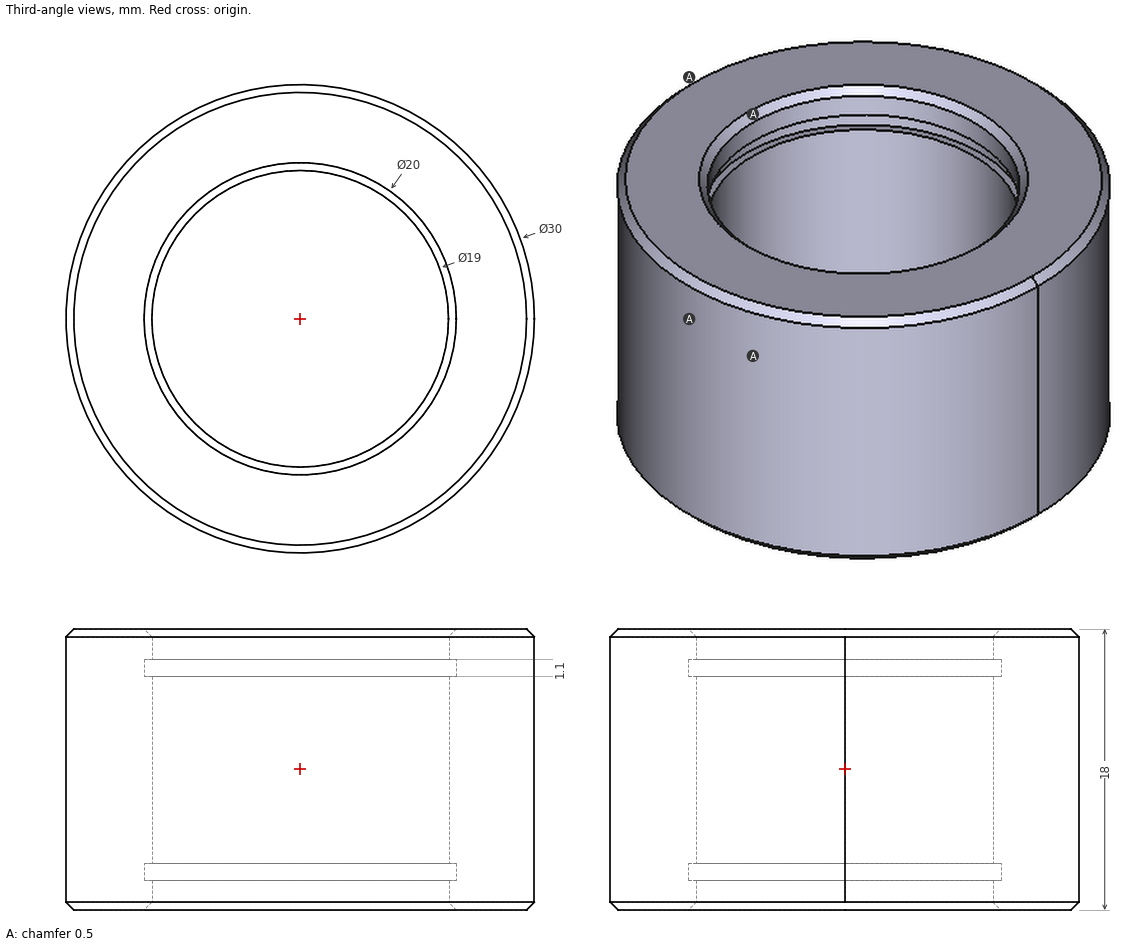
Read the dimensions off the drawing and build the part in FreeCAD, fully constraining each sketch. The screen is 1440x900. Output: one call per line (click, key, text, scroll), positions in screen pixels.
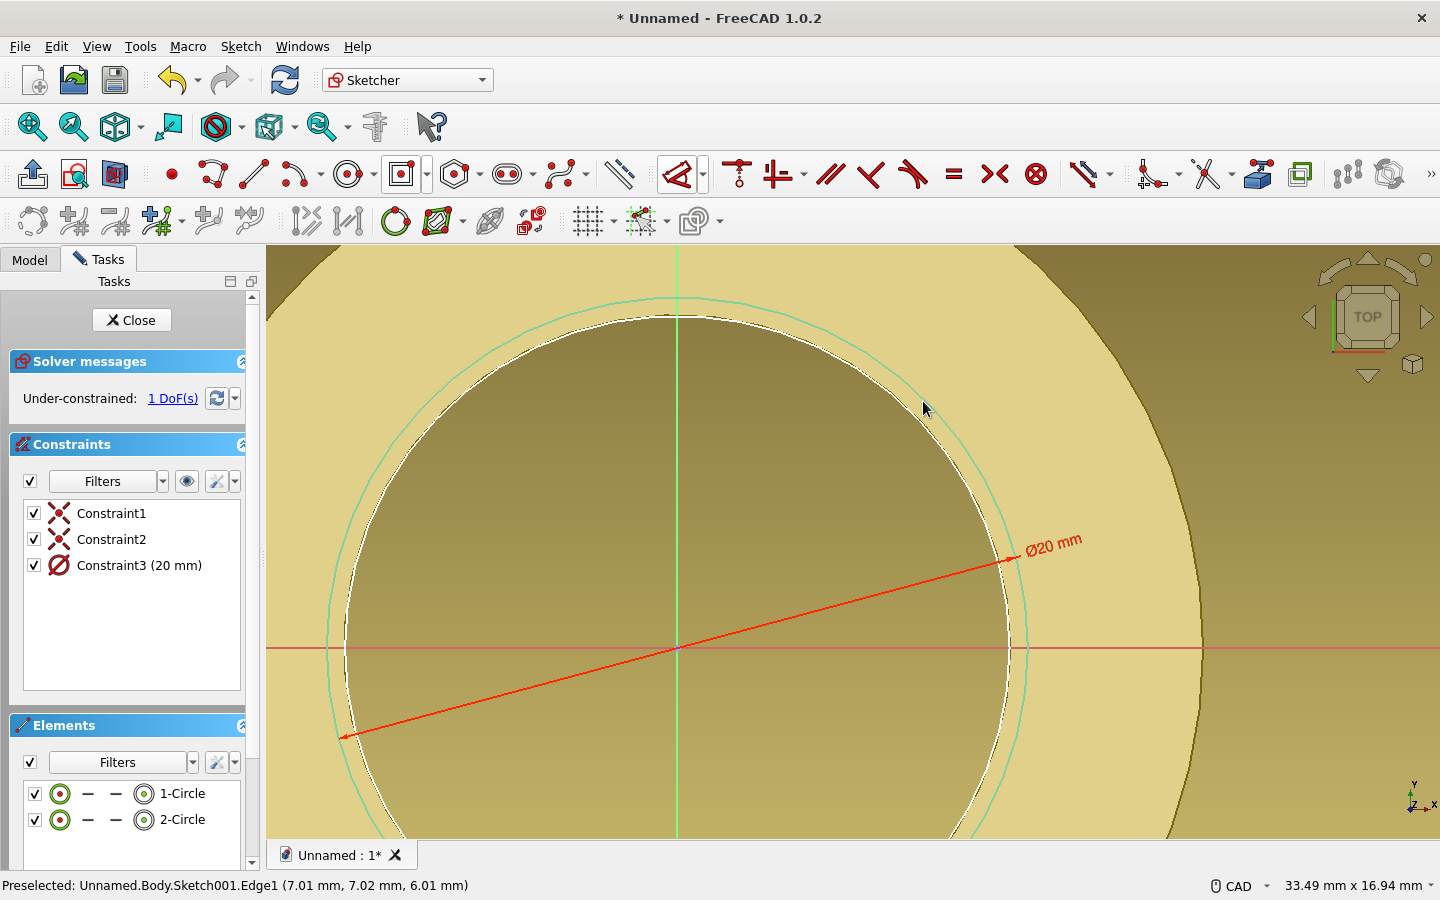
click(912, 413)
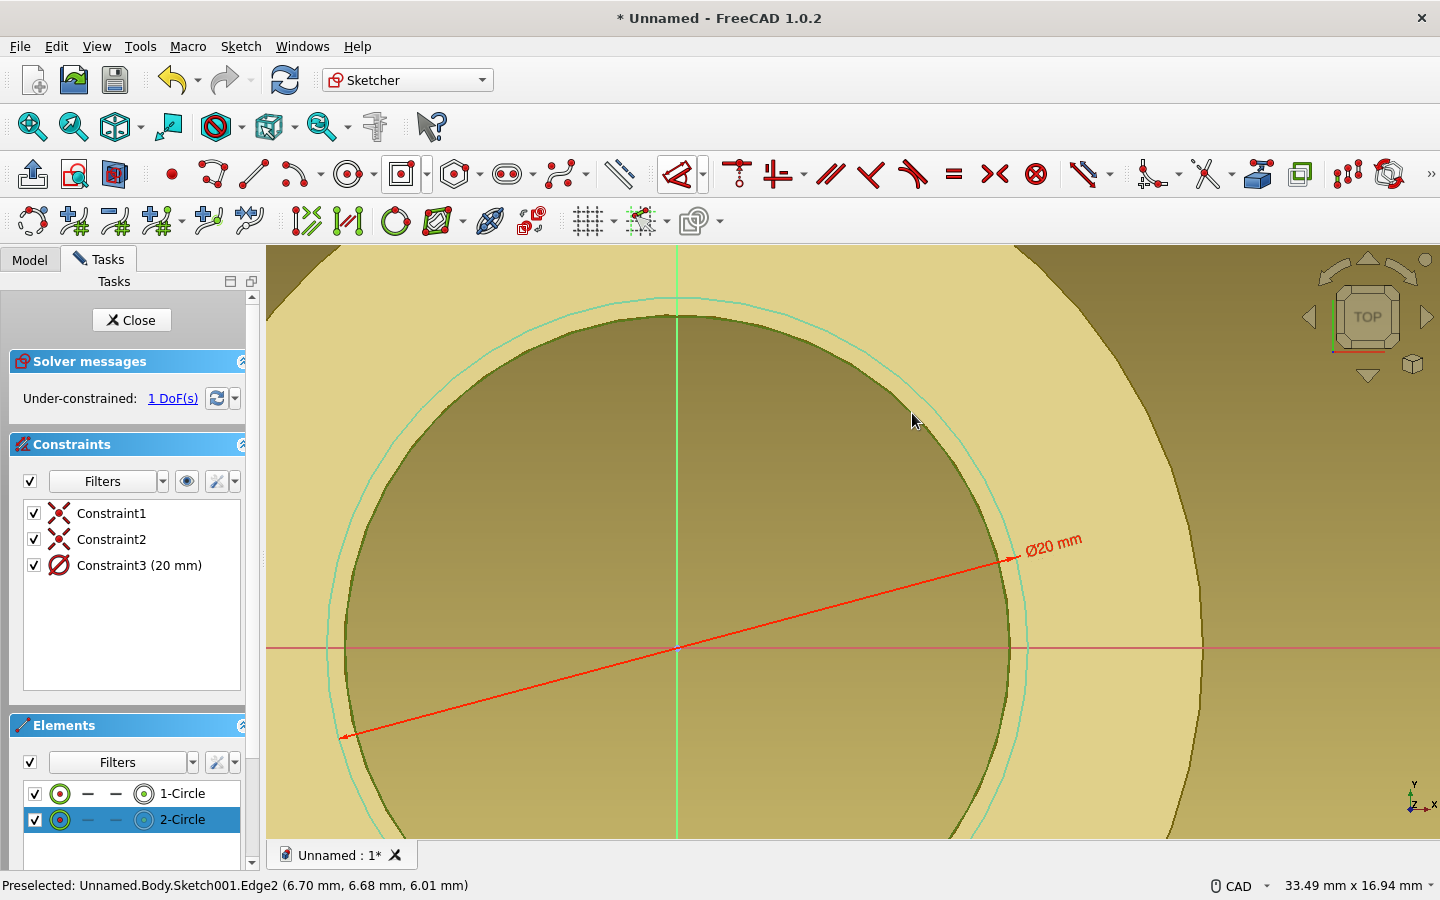
key(k)
key(o)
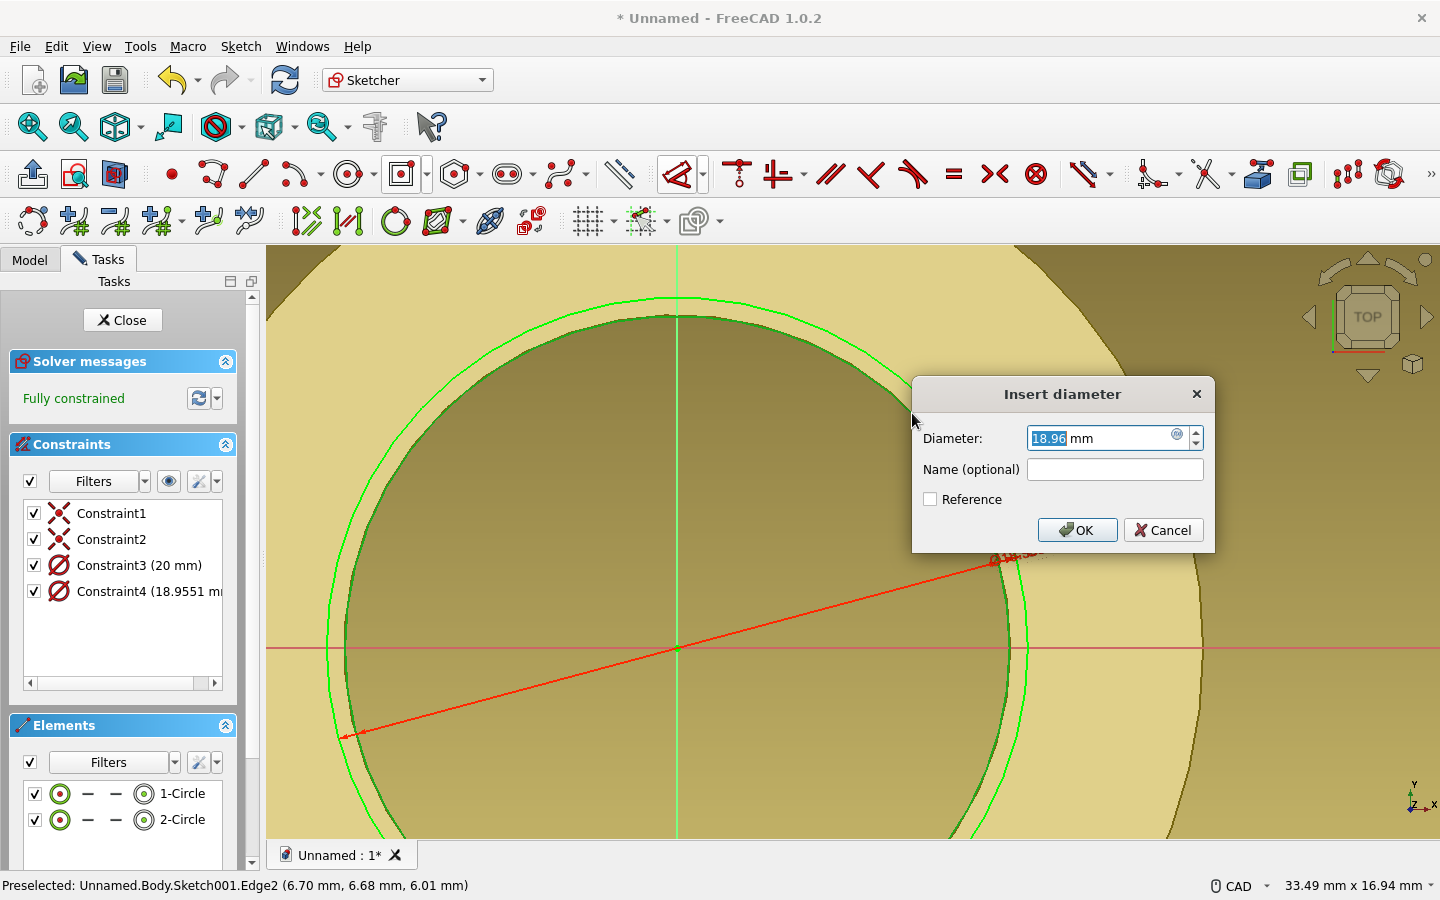
text(19)
key(Return)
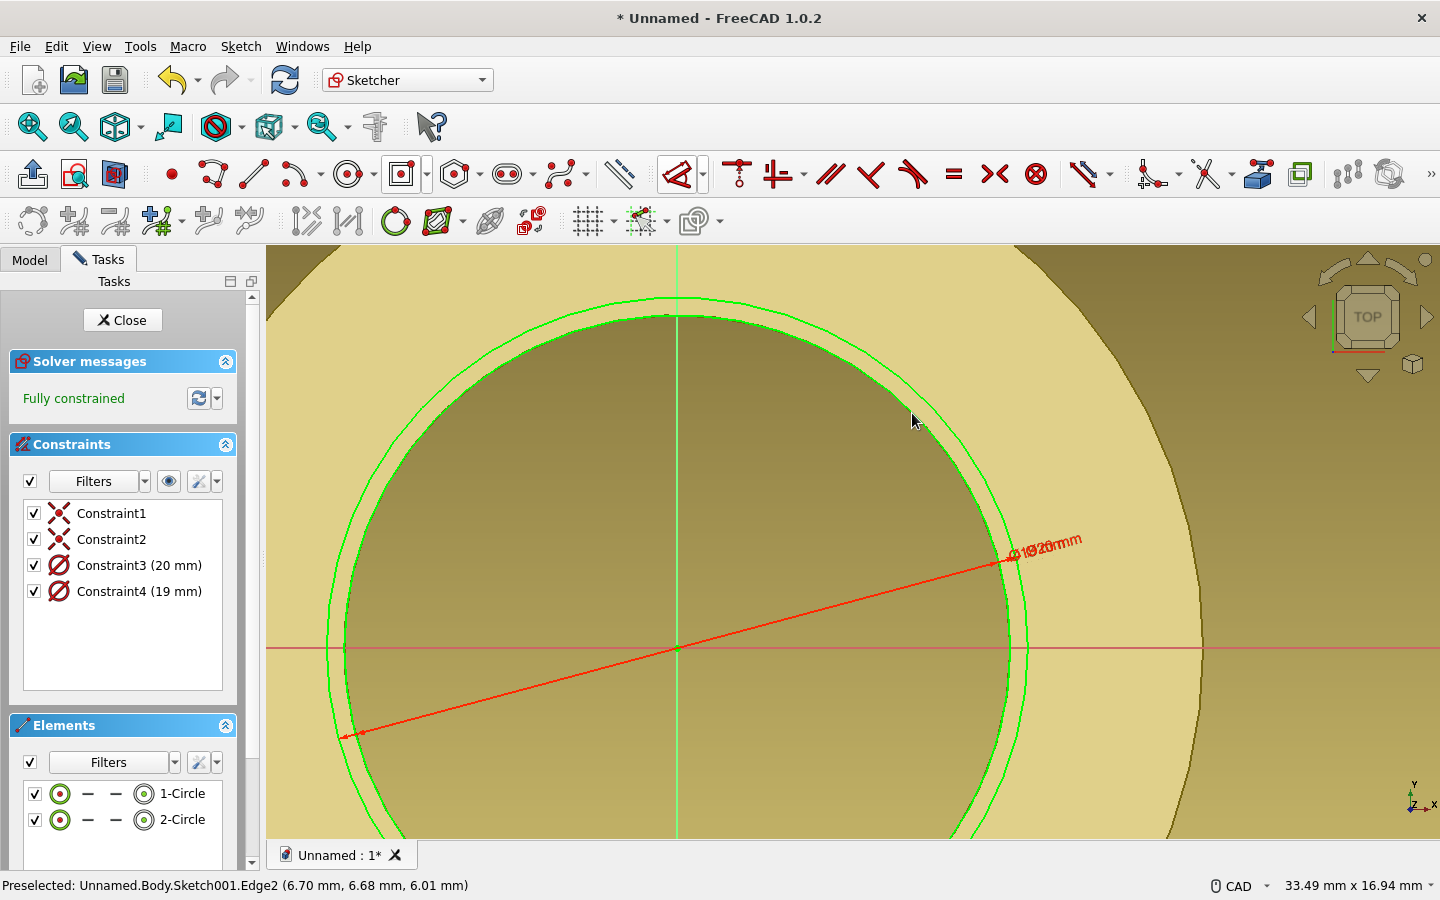
click(123, 320)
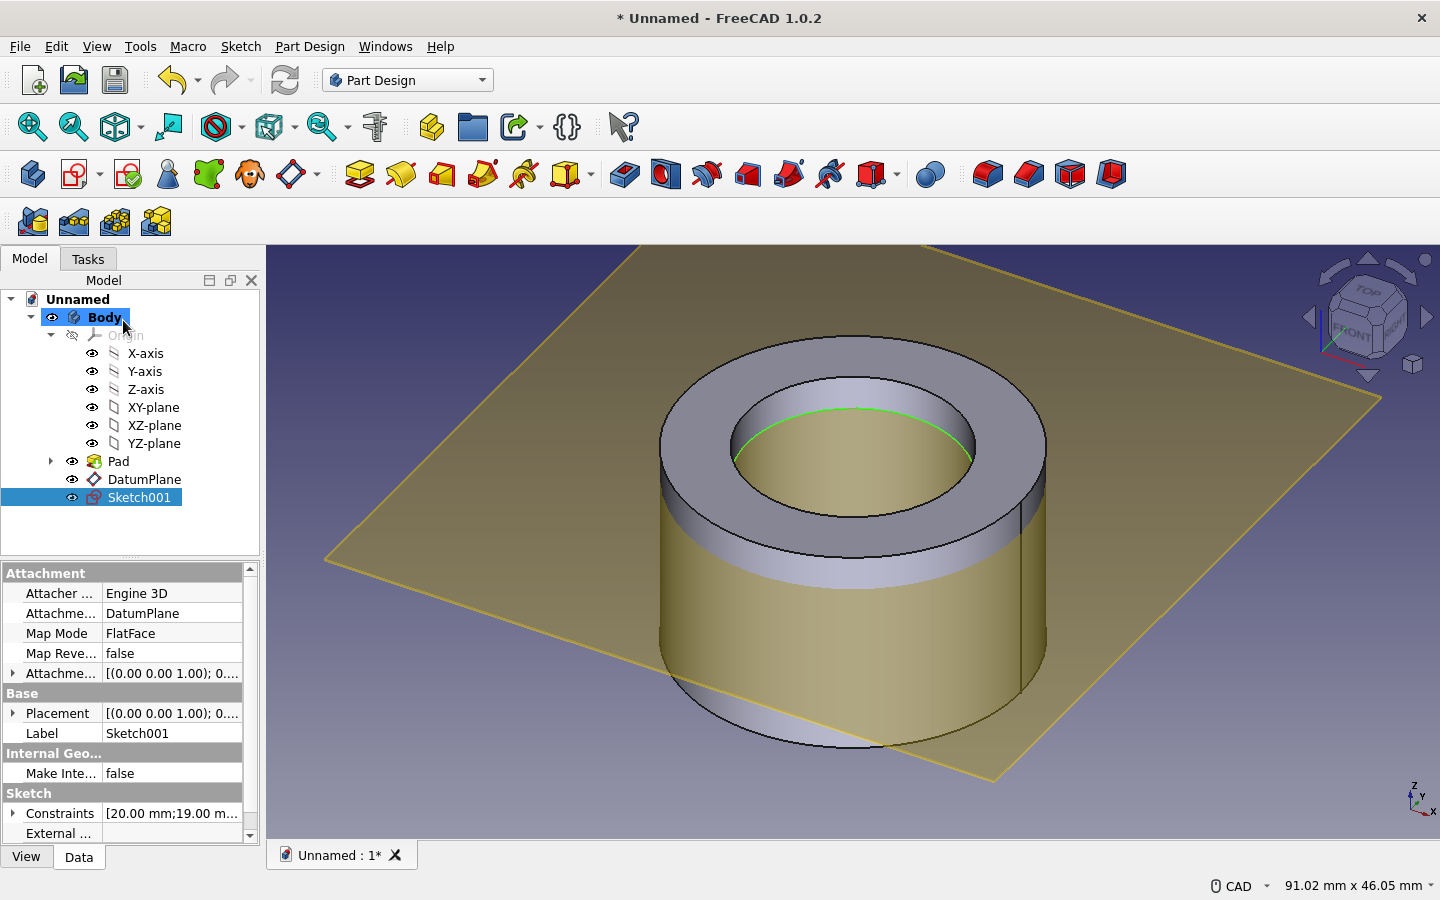
click(625, 174)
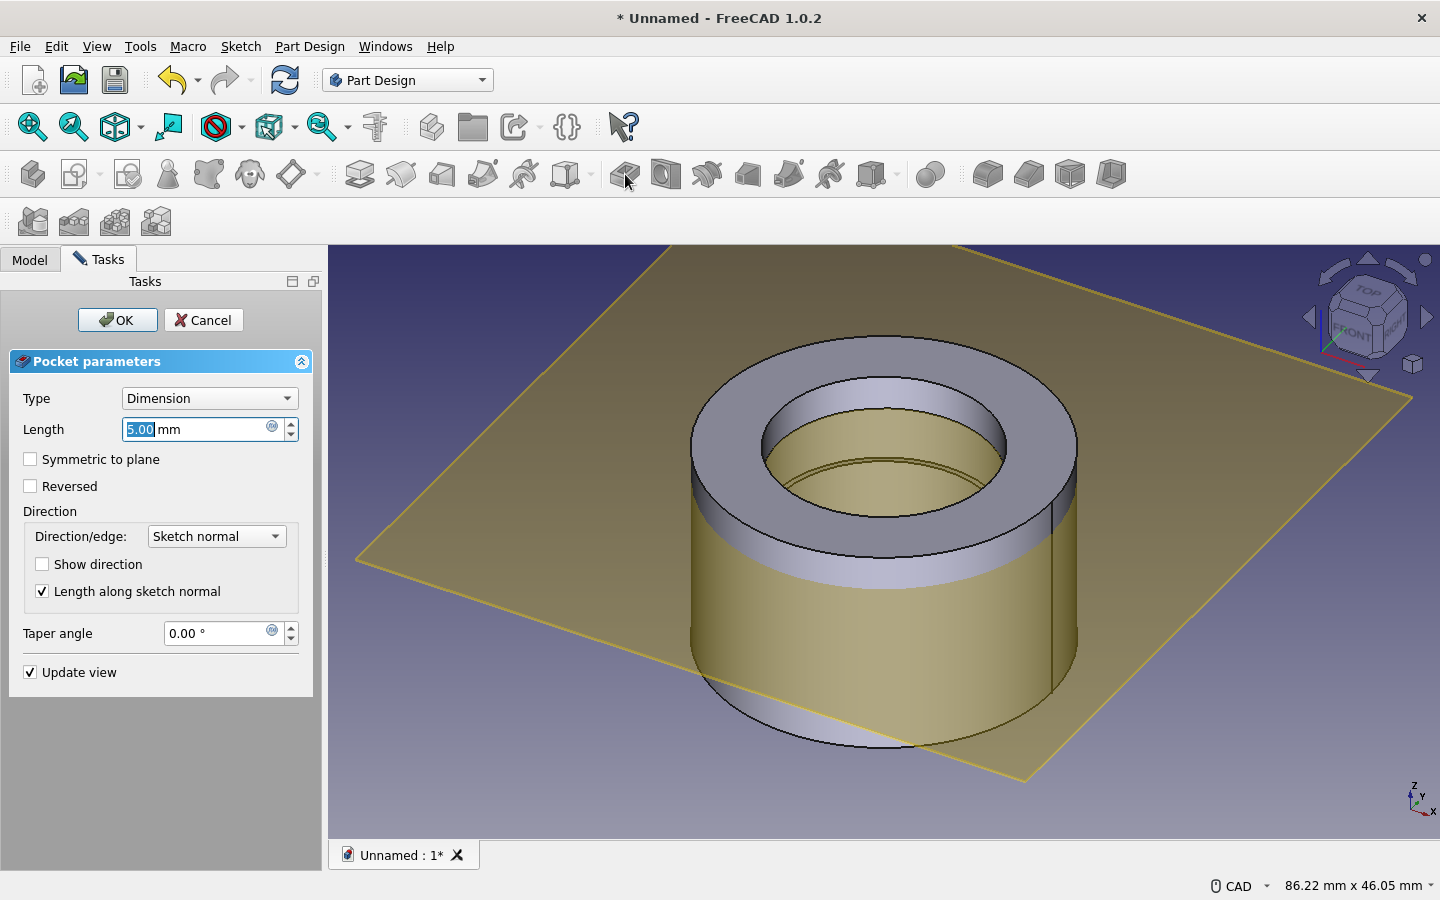
text(1.1)
key(Tab)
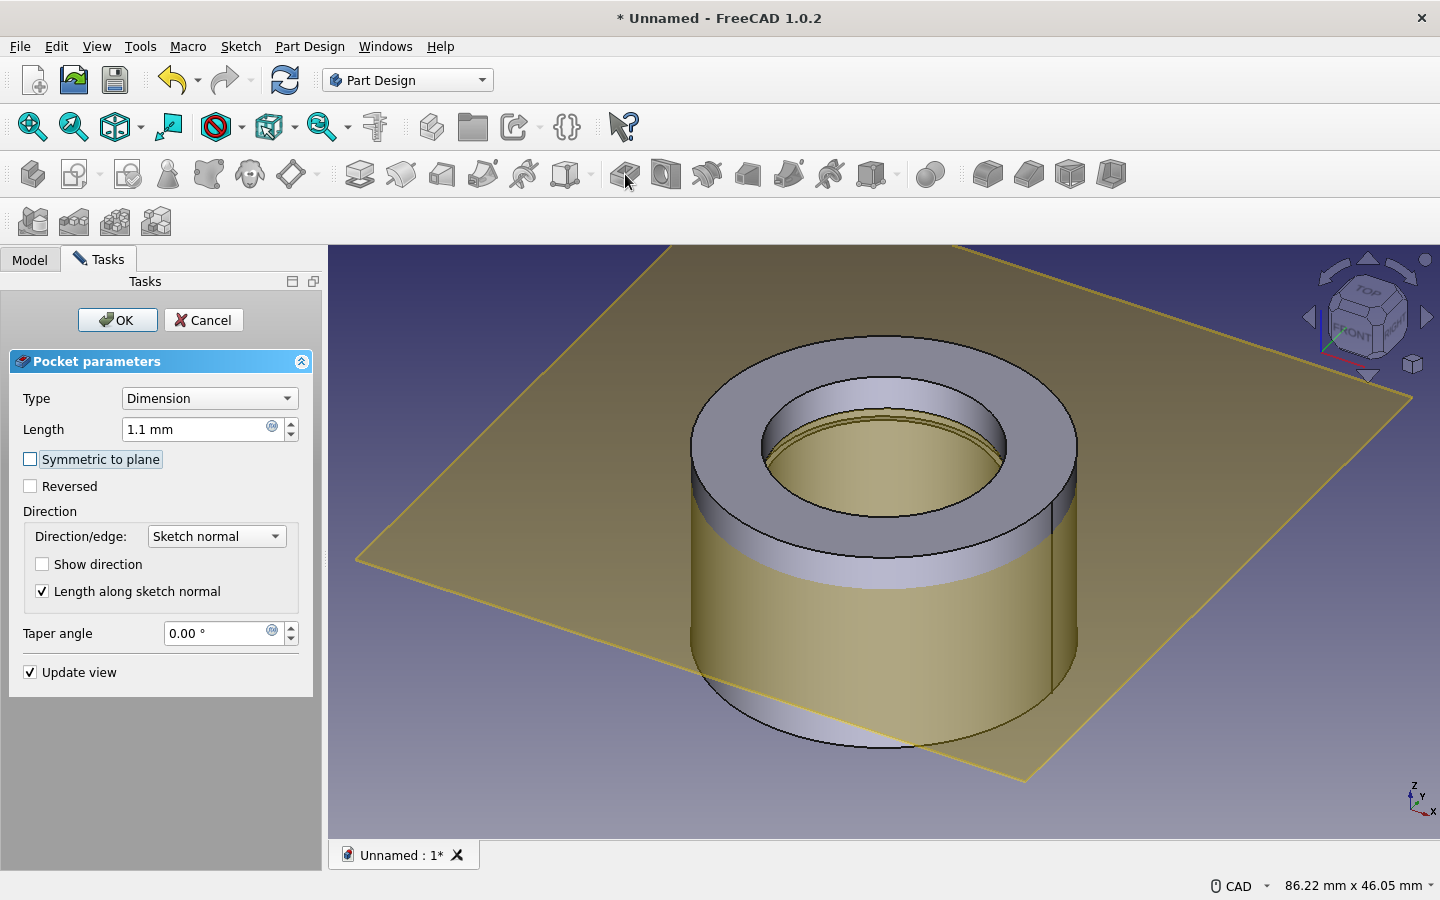
click(31, 486)